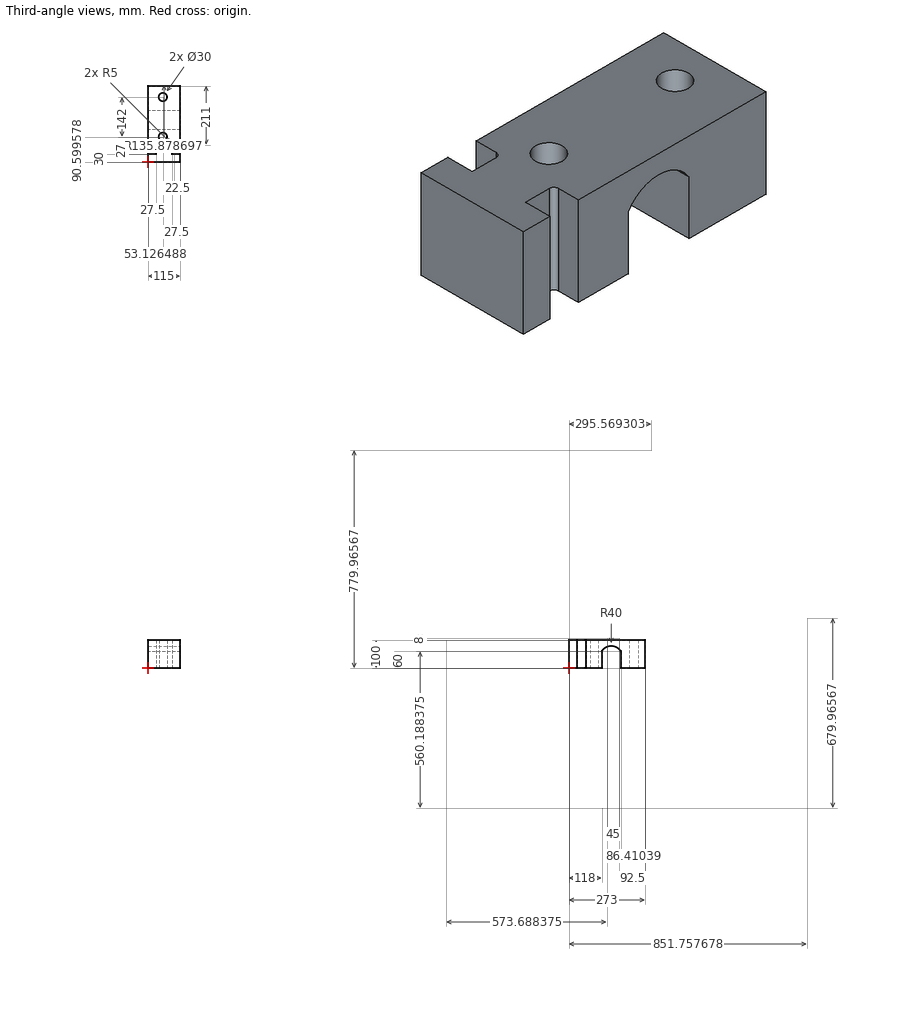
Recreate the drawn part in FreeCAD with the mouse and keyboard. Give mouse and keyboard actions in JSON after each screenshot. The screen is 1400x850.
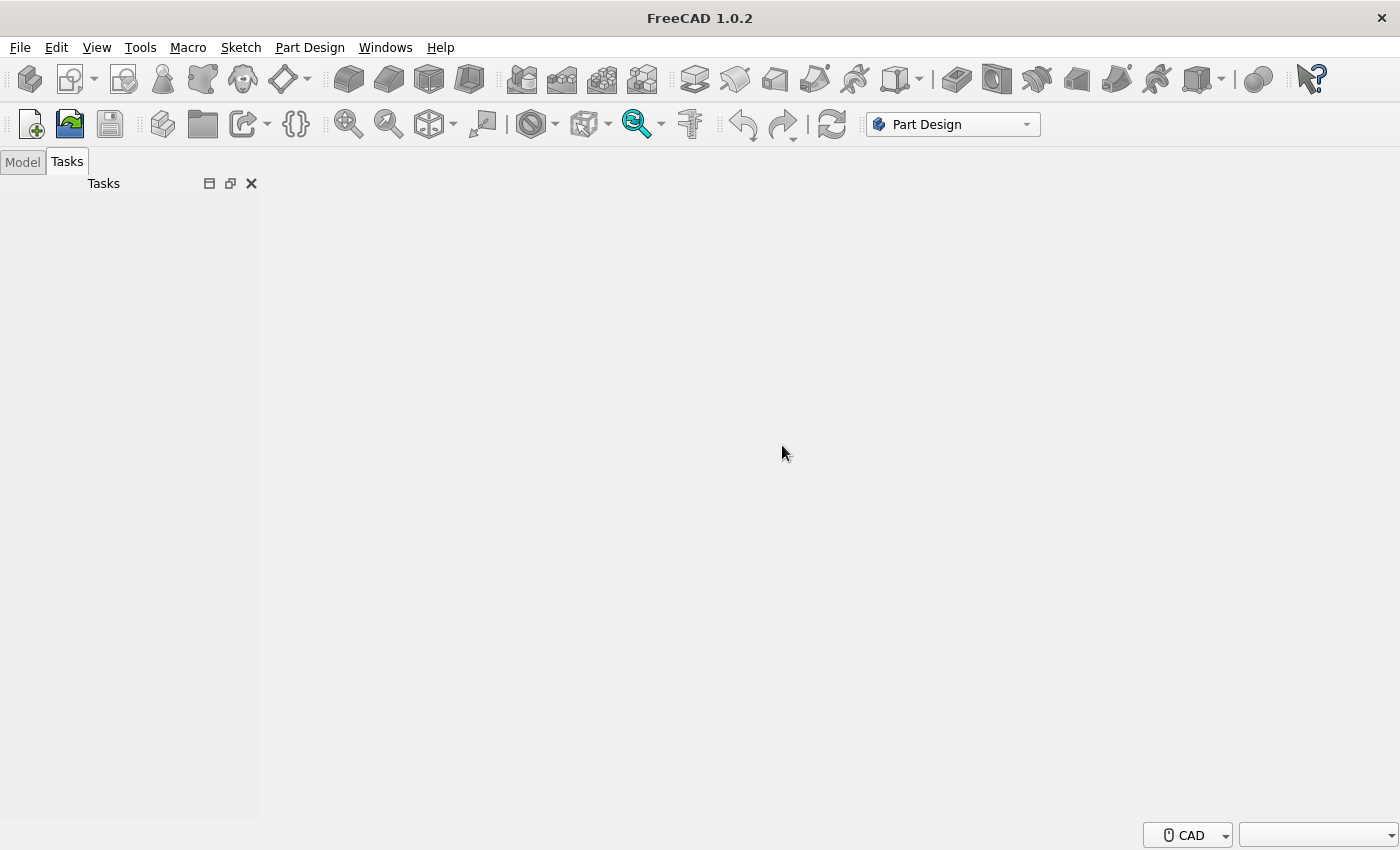
{"action": "key", "text": "ctrl+n"}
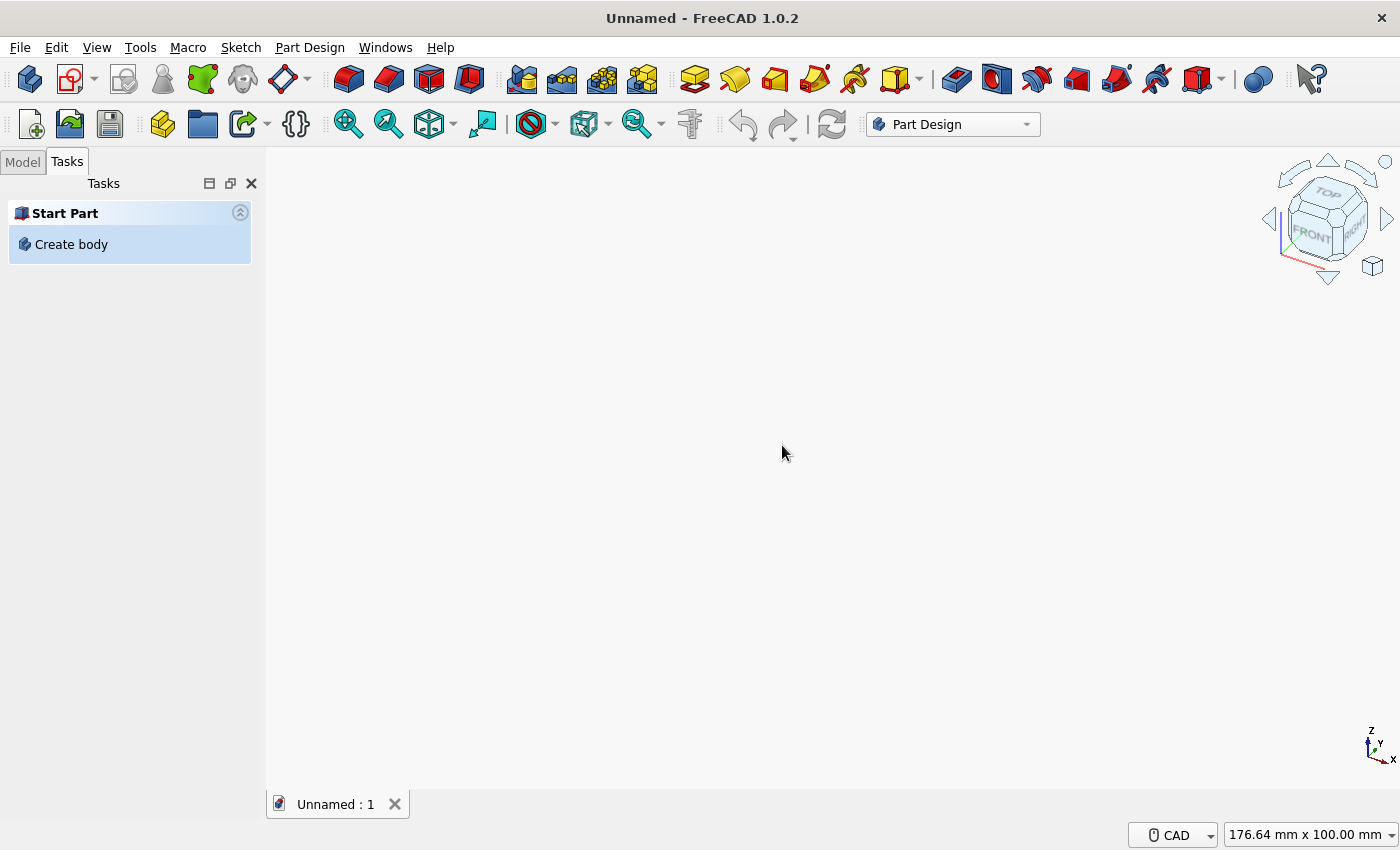
{"action": "left_click", "coordinate": [70, 80]}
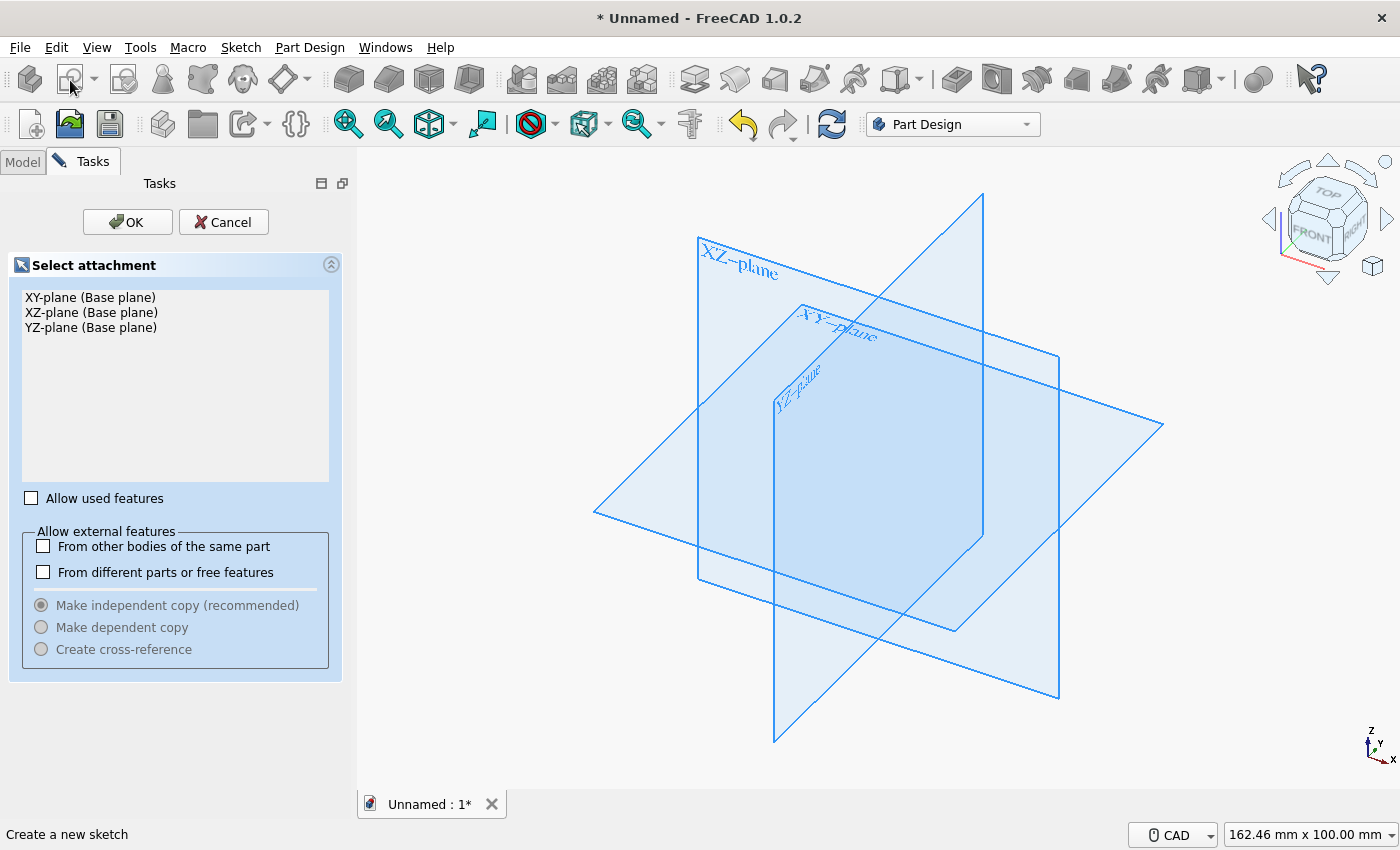
{"action": "left_click", "coordinate": [82, 298]}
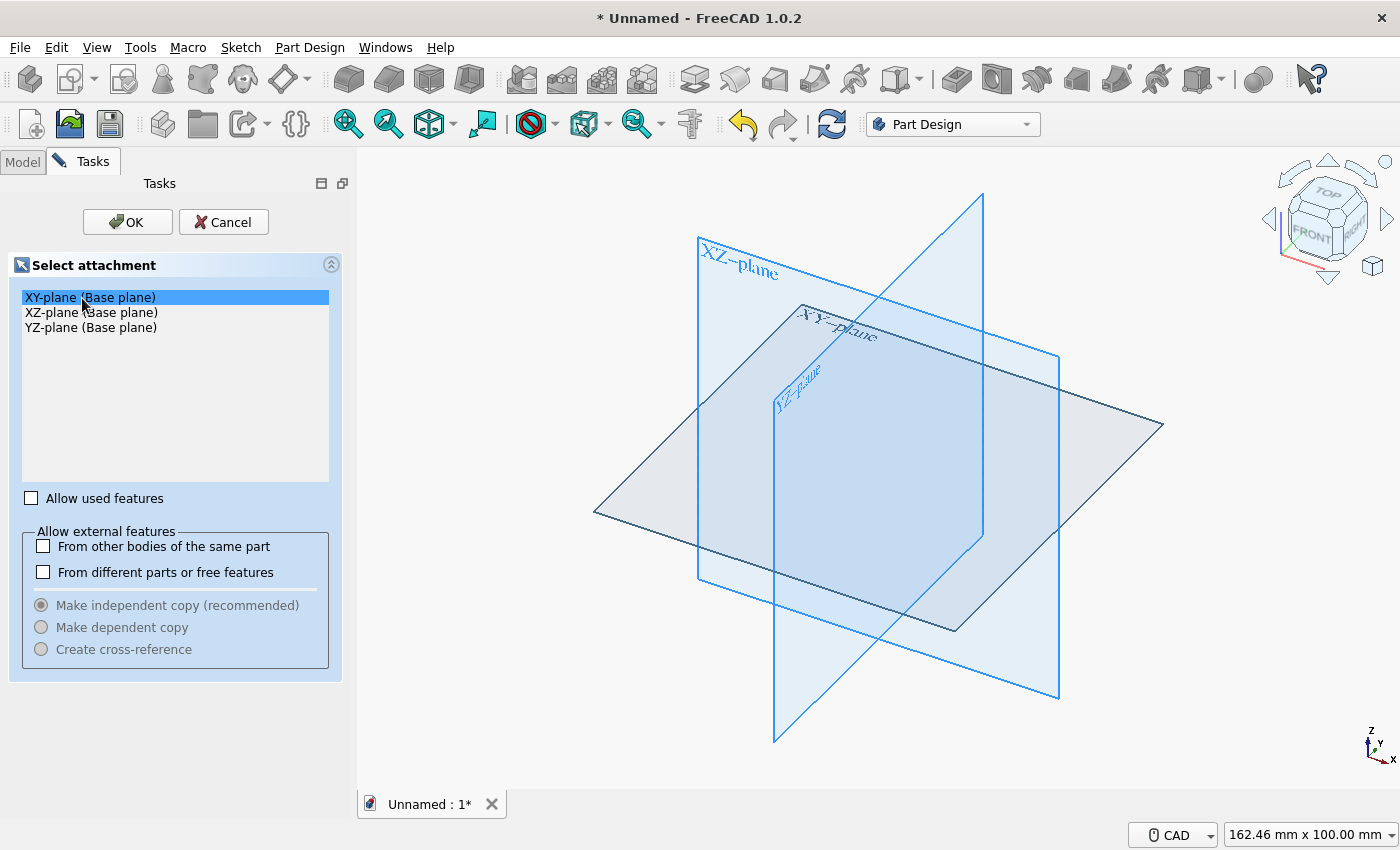
{"action": "left_click", "coordinate": [128, 222]}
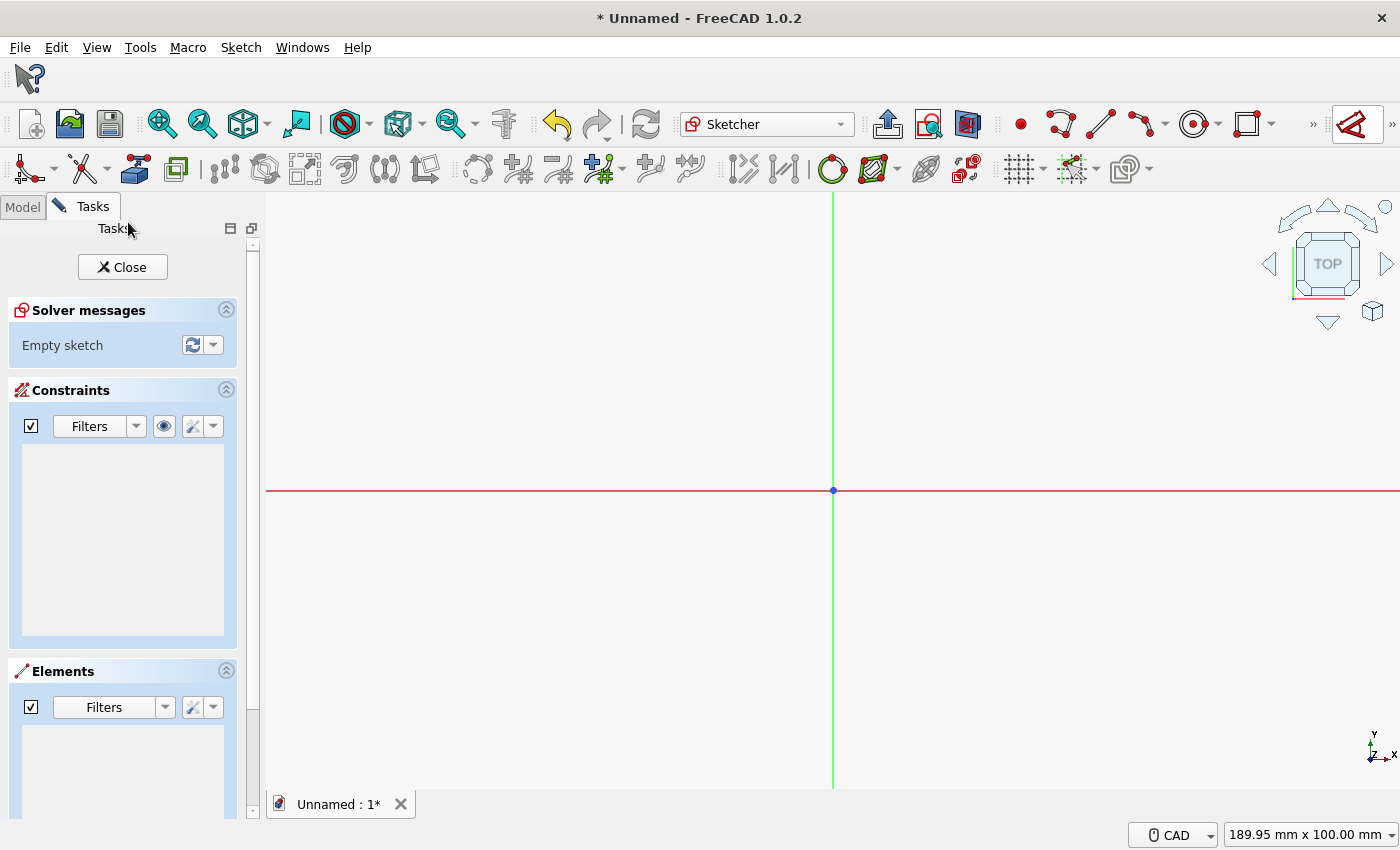
{"action": "scroll", "coordinate": [630, 761], "scroll_direction": "down", "scroll_amount": 7}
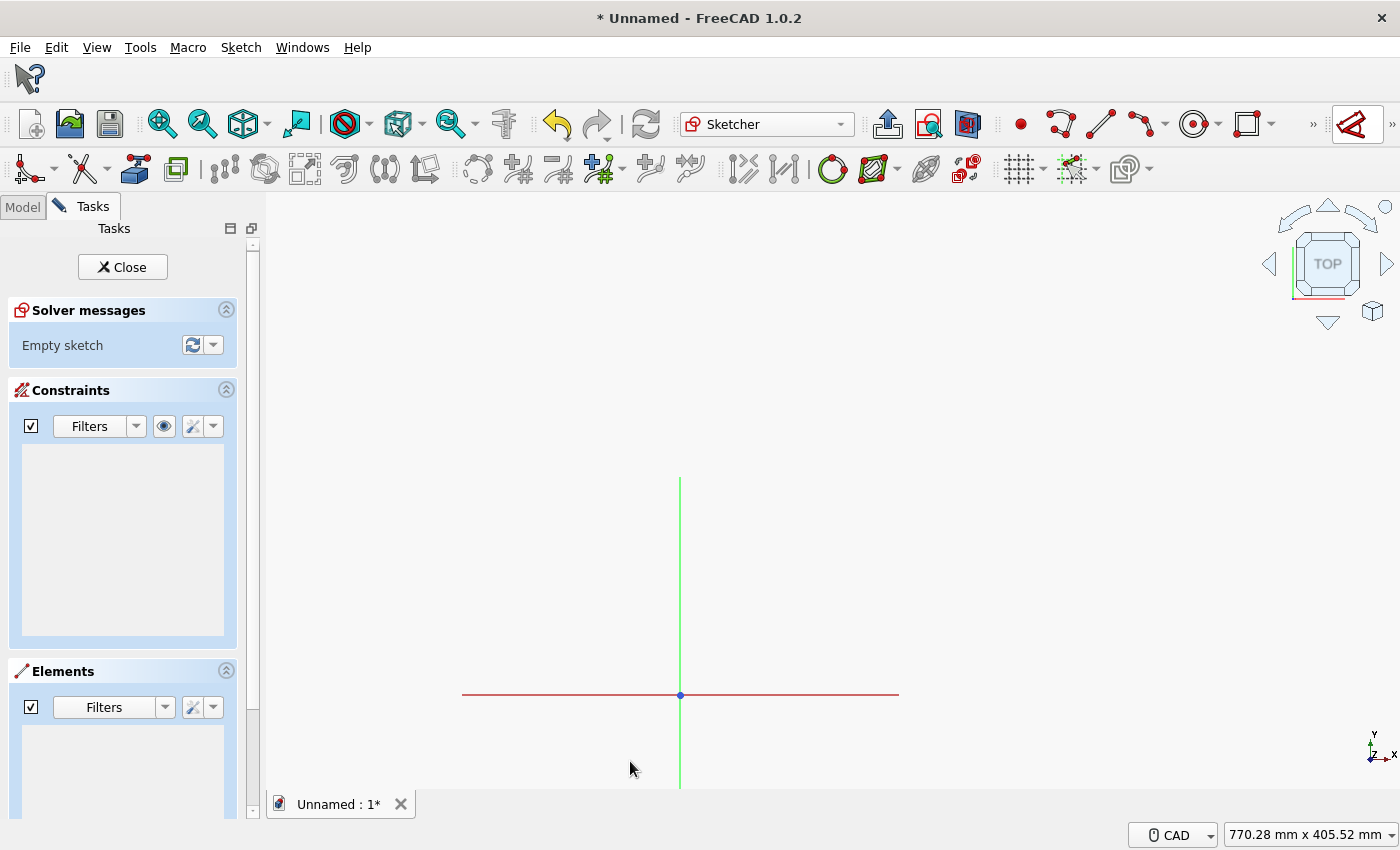
{"action": "key", "text": "g m"}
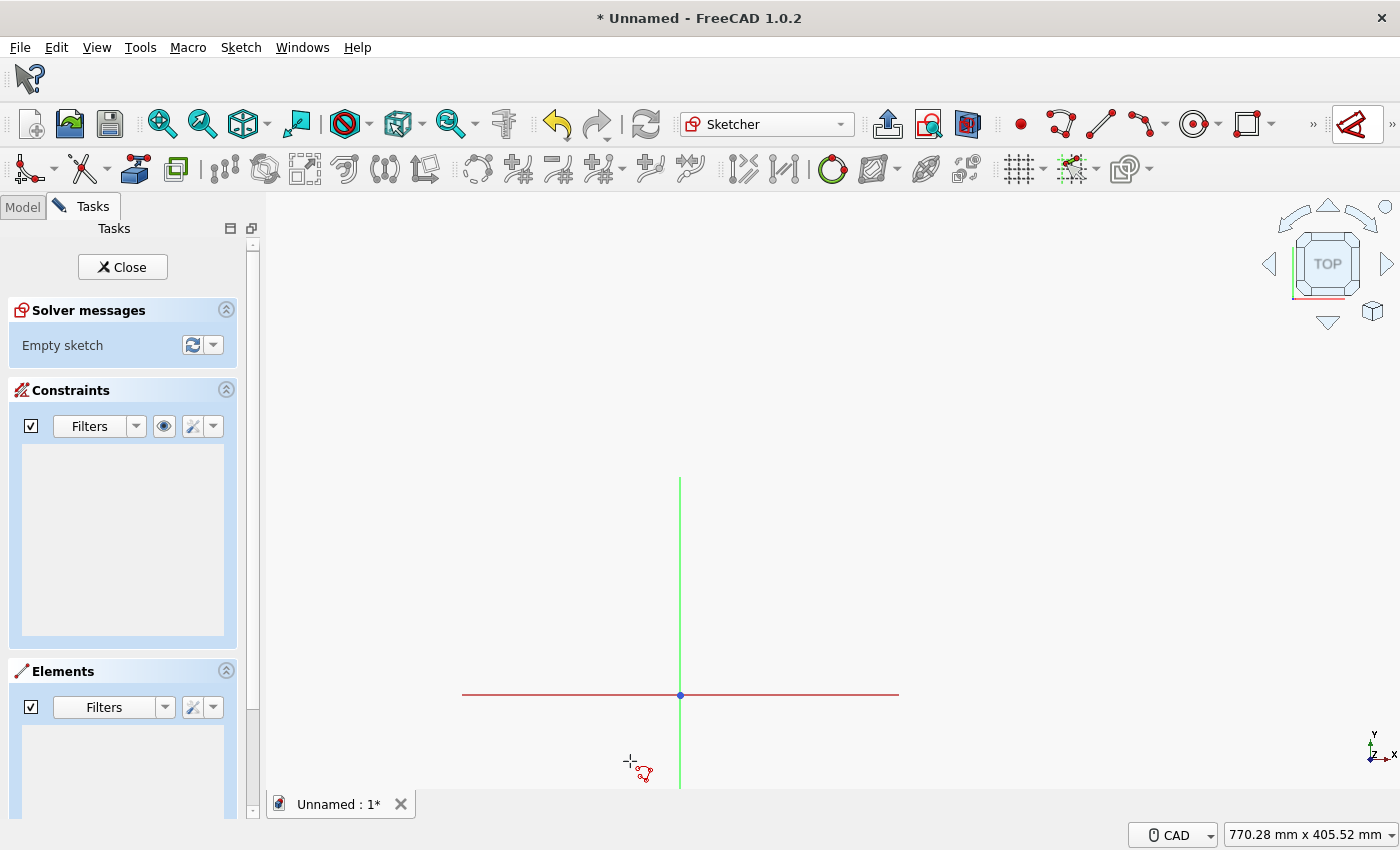
{"action": "left_click", "coordinate": [721, 611]}
{"action": "left_click", "coordinate": [721, 651]}
{"action": "left_click", "coordinate": [680, 651]}
{"action": "left_click", "coordinate": [680, 695]}
{"action": "left_click", "coordinate": [850, 686]}
{"action": "left_click", "coordinate": [850, 651]}
{"action": "left_click", "coordinate": [809, 651]}
{"action": "left_click", "coordinate": [809, 611]}
{"action": "right_click", "coordinate": [809, 611]}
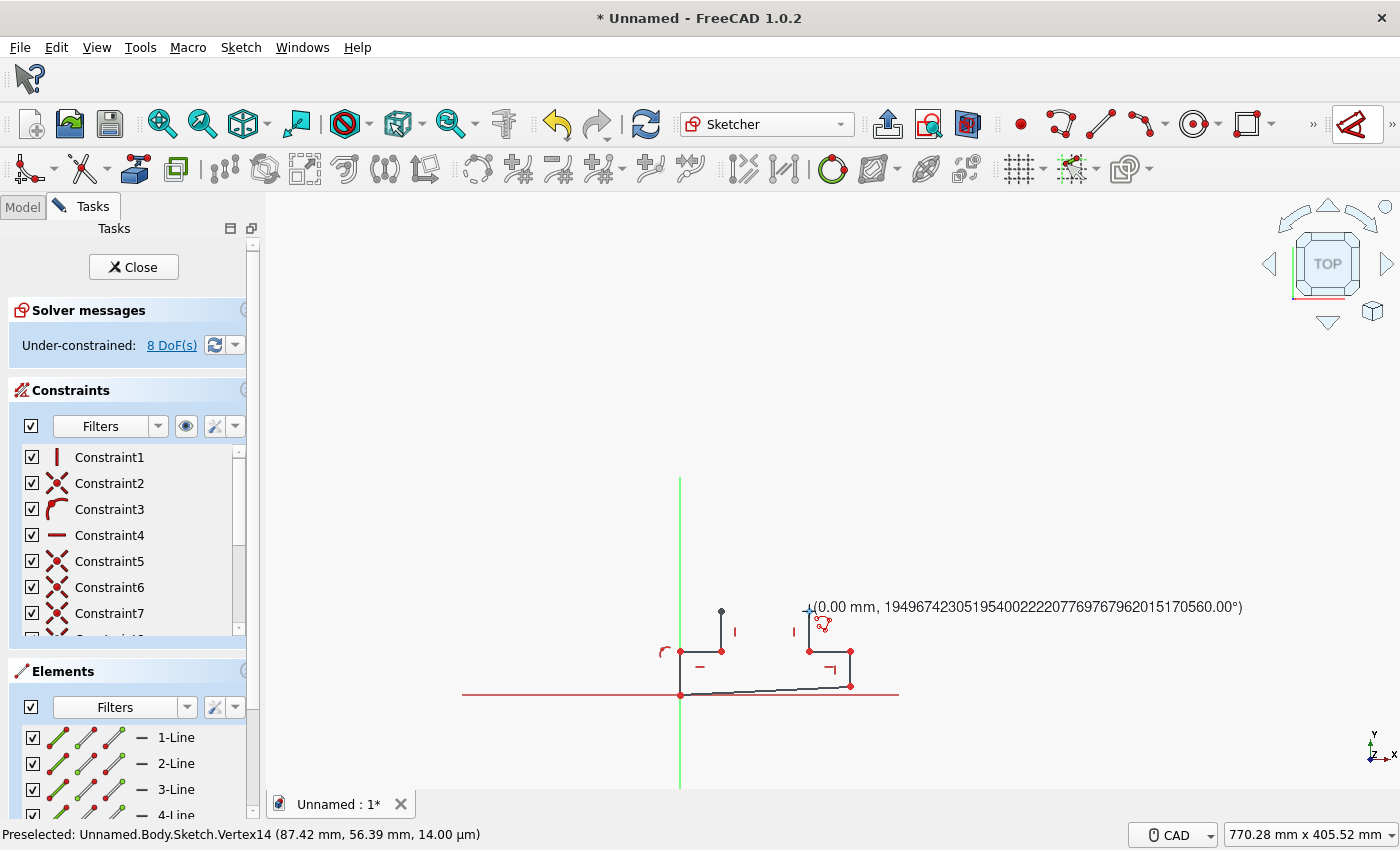
{"action": "scroll", "coordinate": [816, 604], "scroll_direction": "up", "scroll_amount": 3}